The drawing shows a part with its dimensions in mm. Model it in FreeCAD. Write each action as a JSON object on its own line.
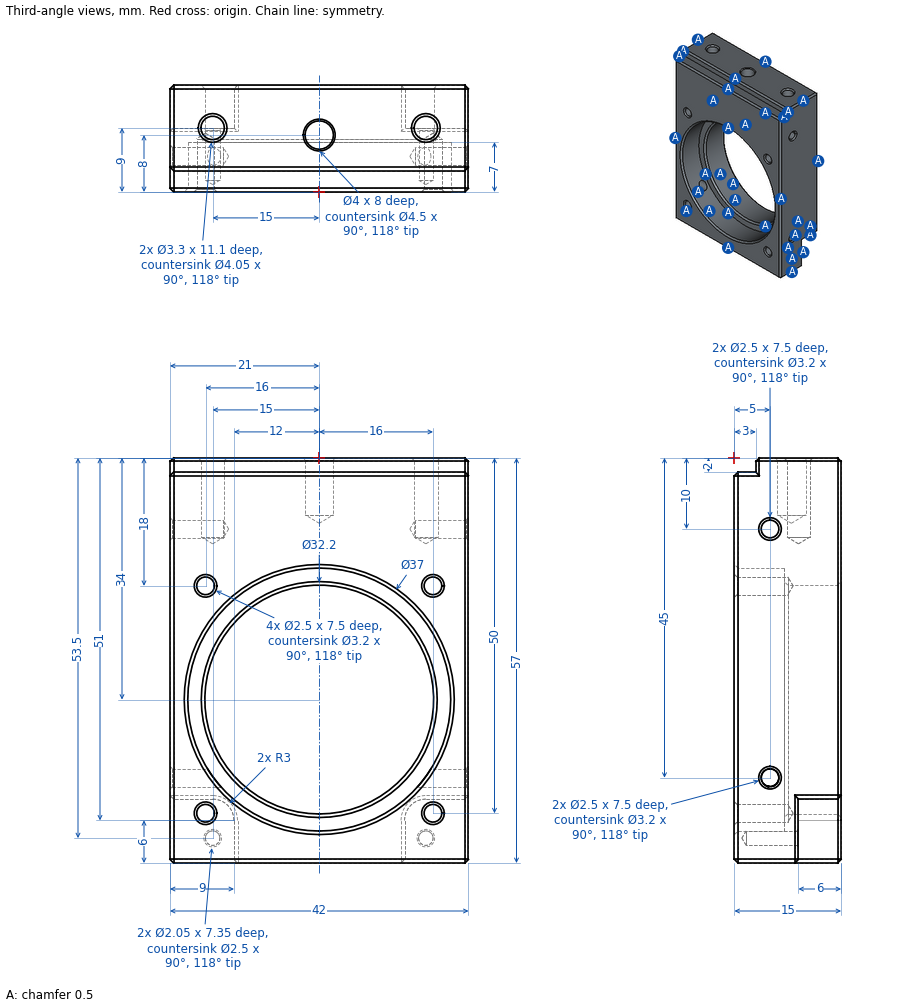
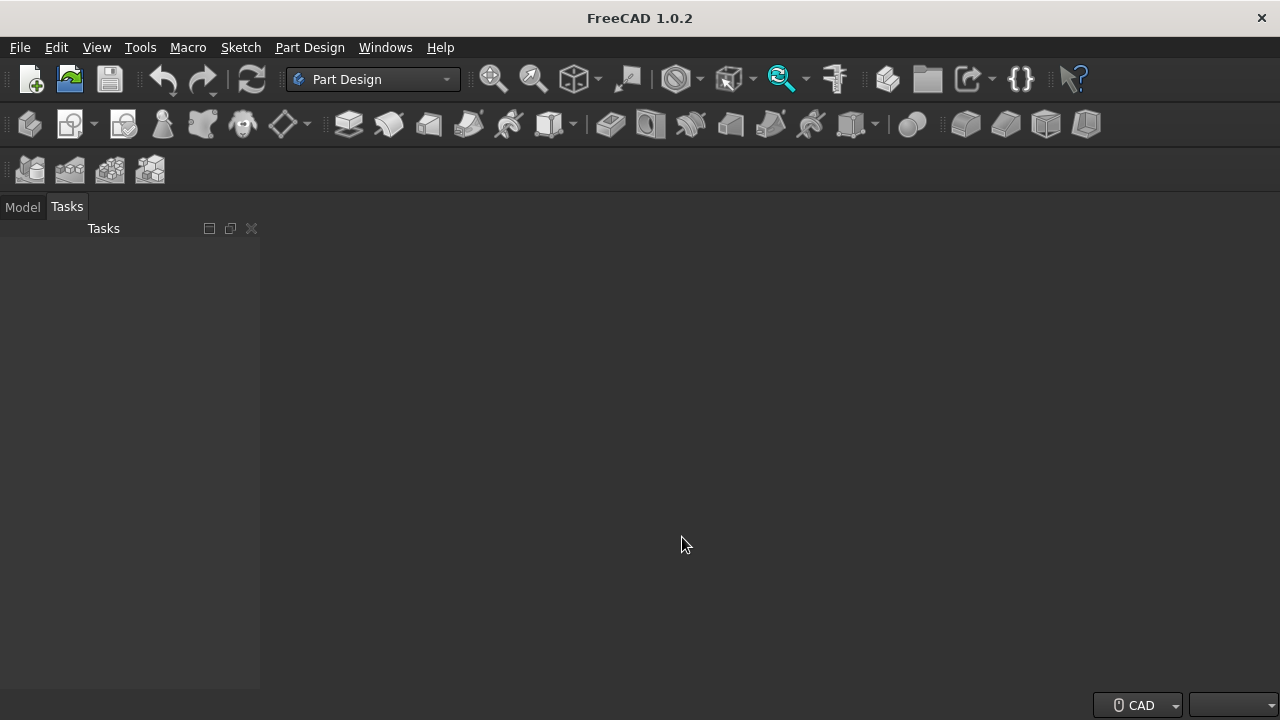
{"action": "key", "text": "ctrl+n"}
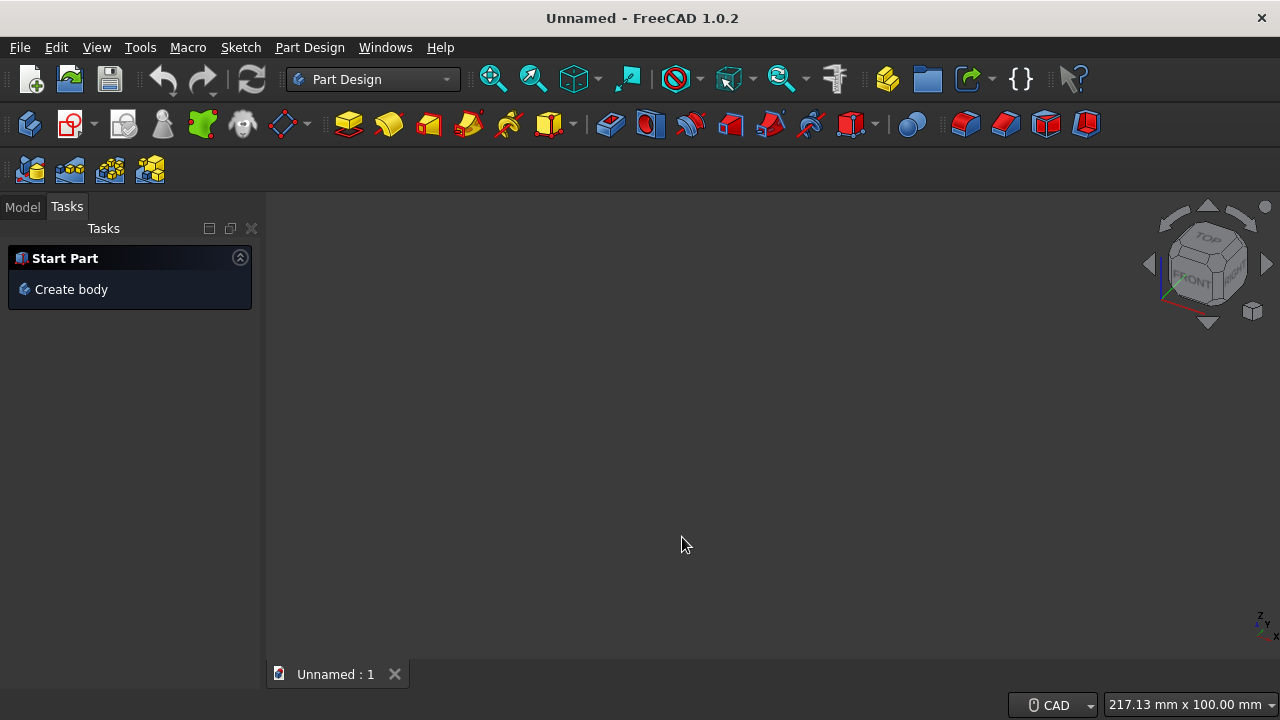
{"action": "left_click", "coordinate": [70, 124]}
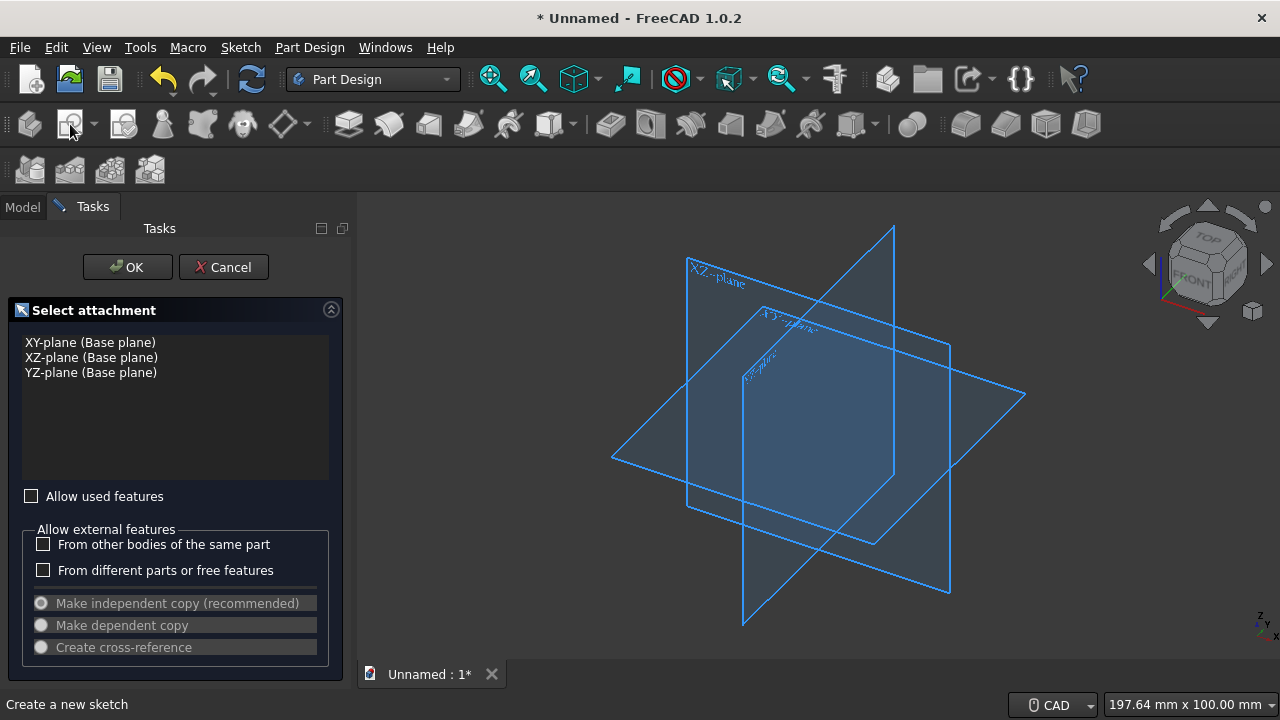
{"action": "left_click", "coordinate": [82, 358]}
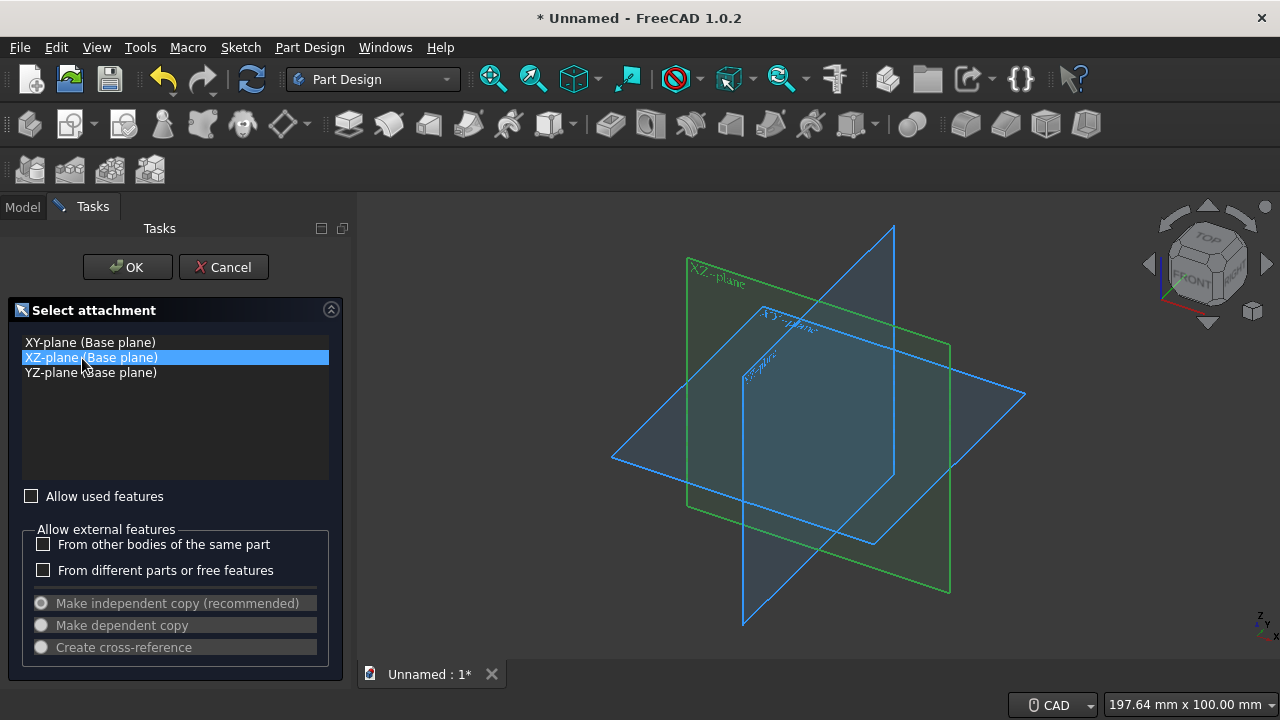
{"action": "left_click", "coordinate": [128, 267]}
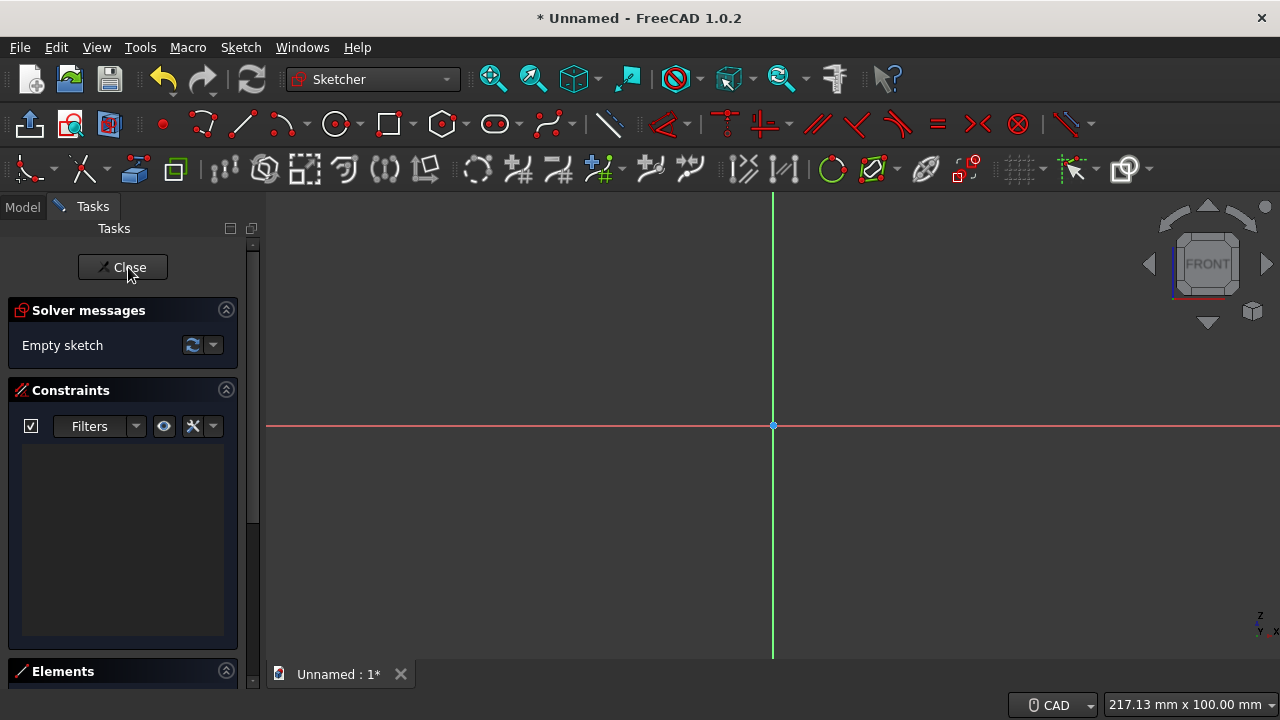
{"action": "scroll", "coordinate": [565, 220], "scroll_direction": "down", "scroll_amount": 2}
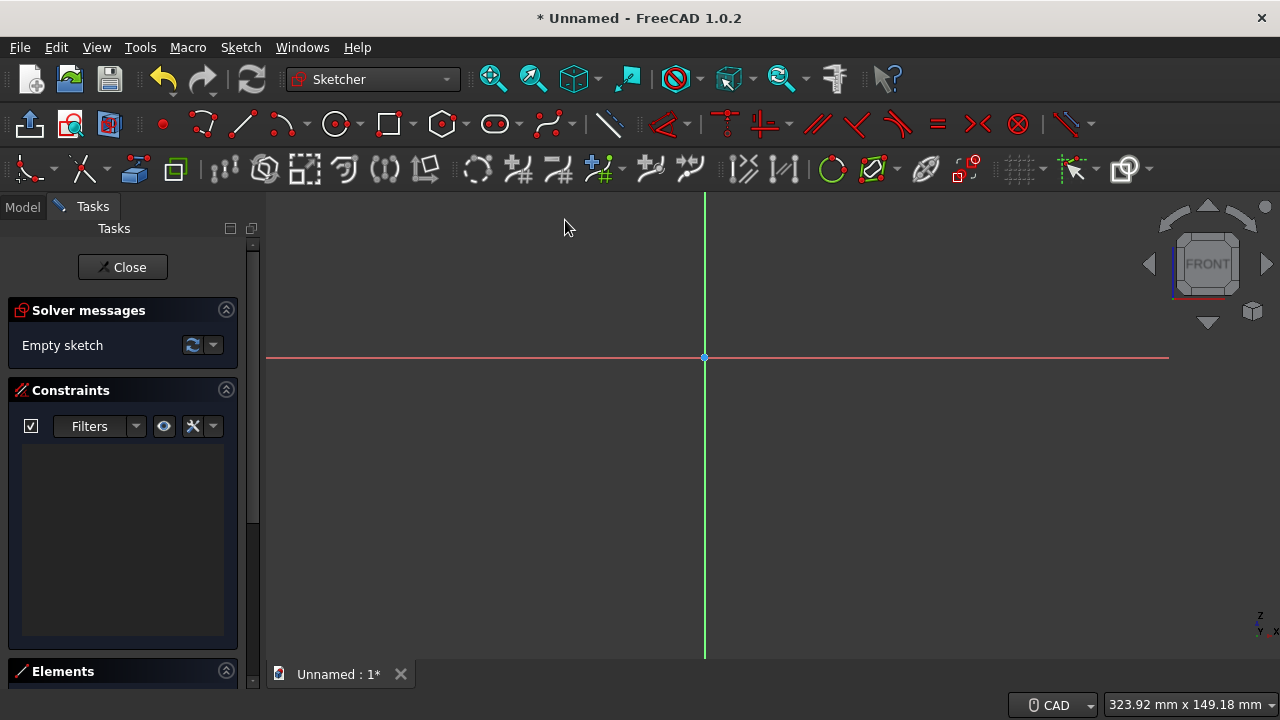
{"action": "scroll", "coordinate": [705, 491], "scroll_direction": "up", "scroll_amount": 2}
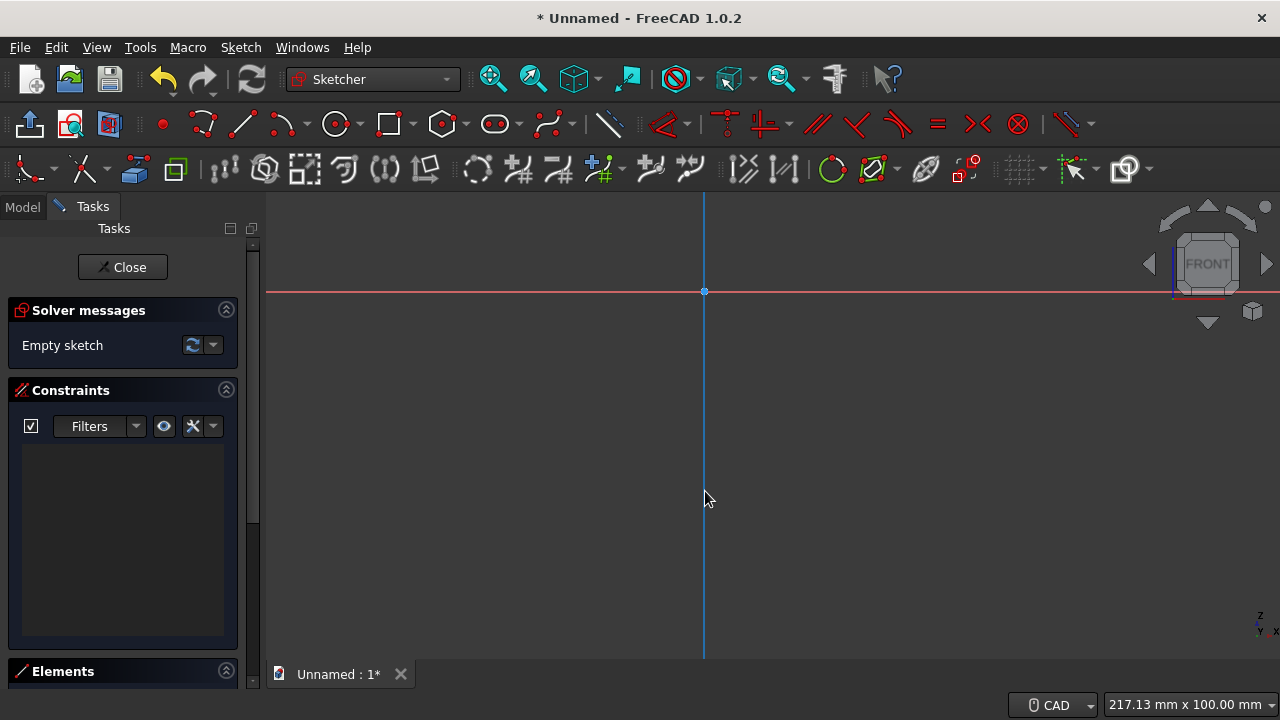
{"action": "left_click", "coordinate": [390, 124]}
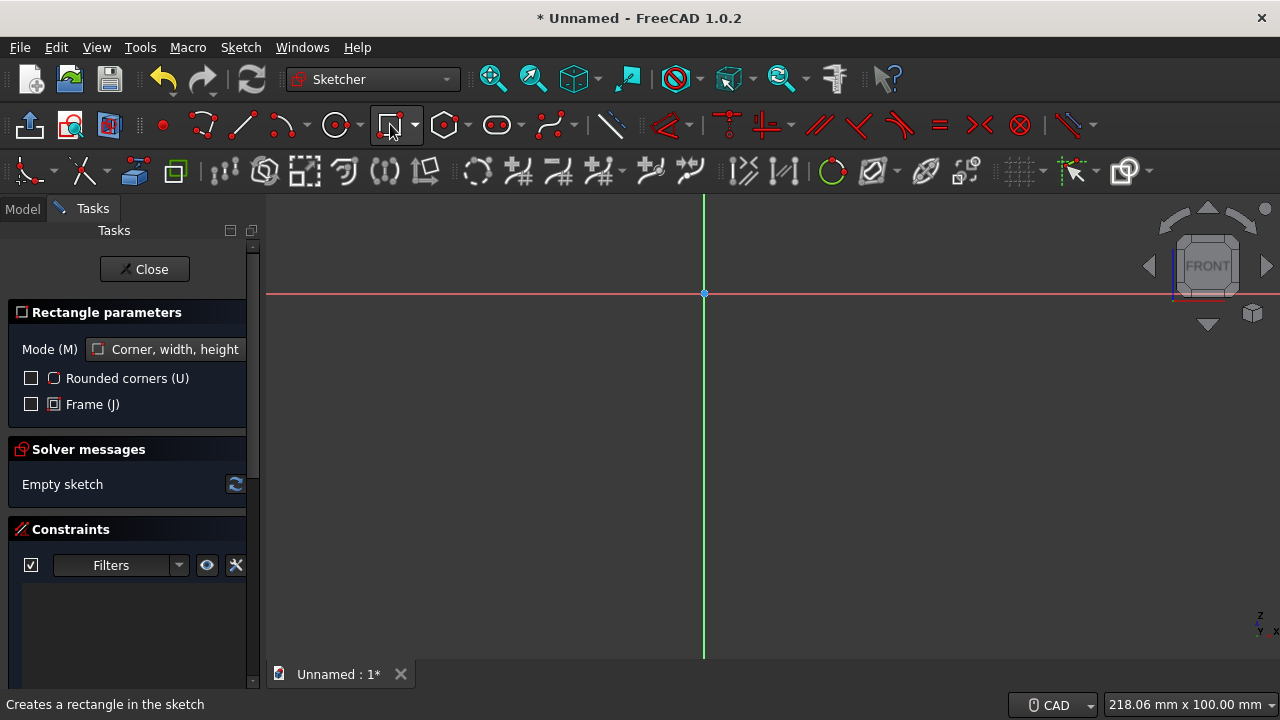
{"action": "left_click", "coordinate": [607, 294]}
{"action": "mouse_move", "coordinate": [802, 559]}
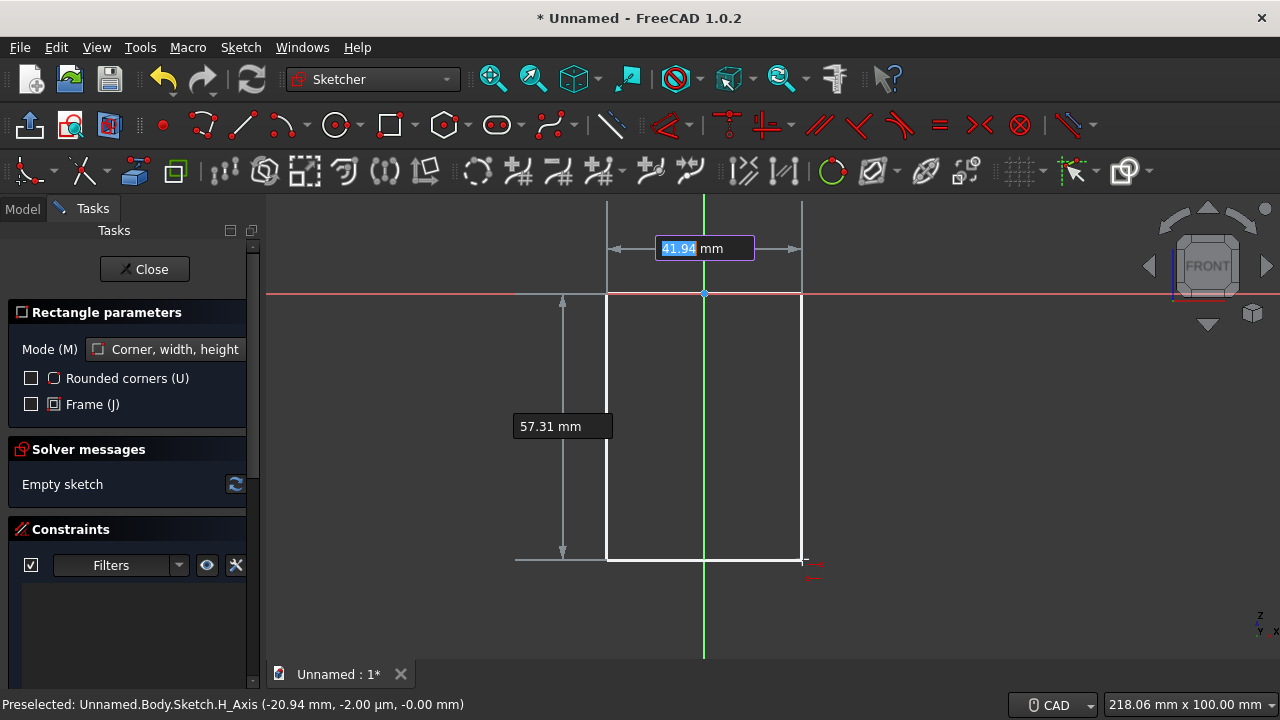
{"action": "type", "text": "42"}
{"action": "key", "text": "Tab"}
{"action": "type", "text": "57"}
{"action": "key", "text": "Return"}
{"action": "key", "text": "Escape"}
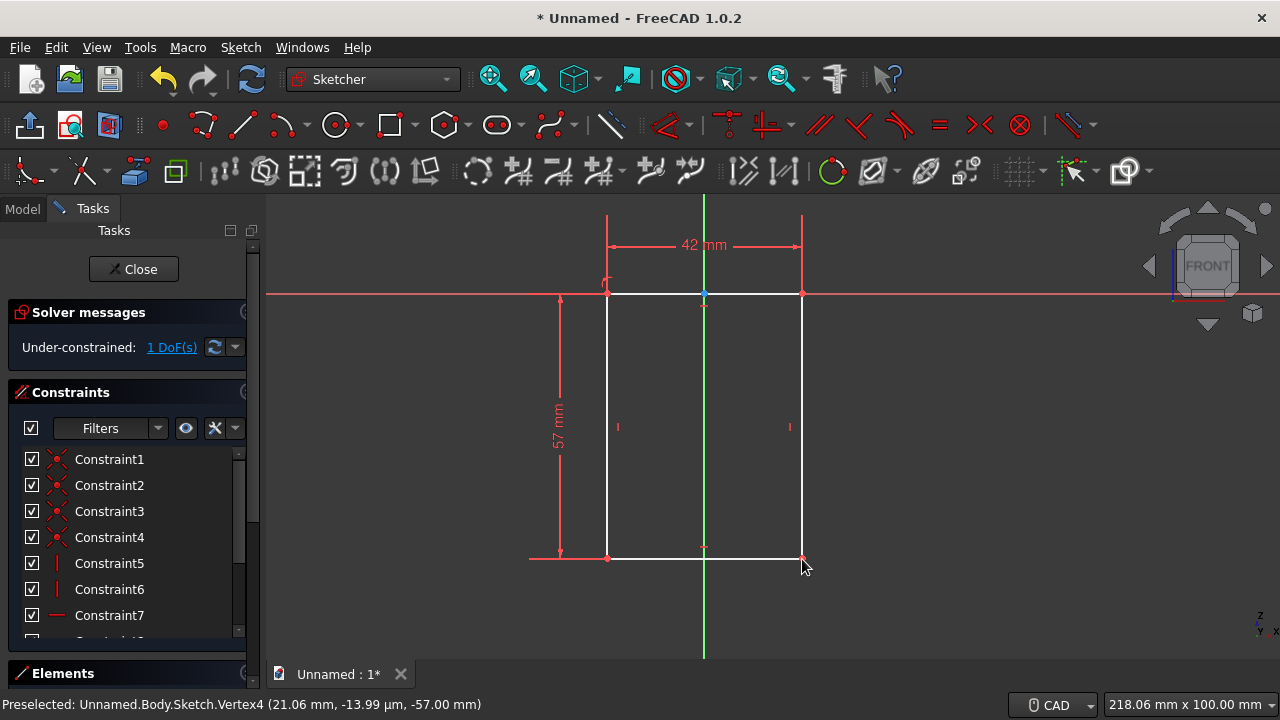
{"action": "key", "text": "d"}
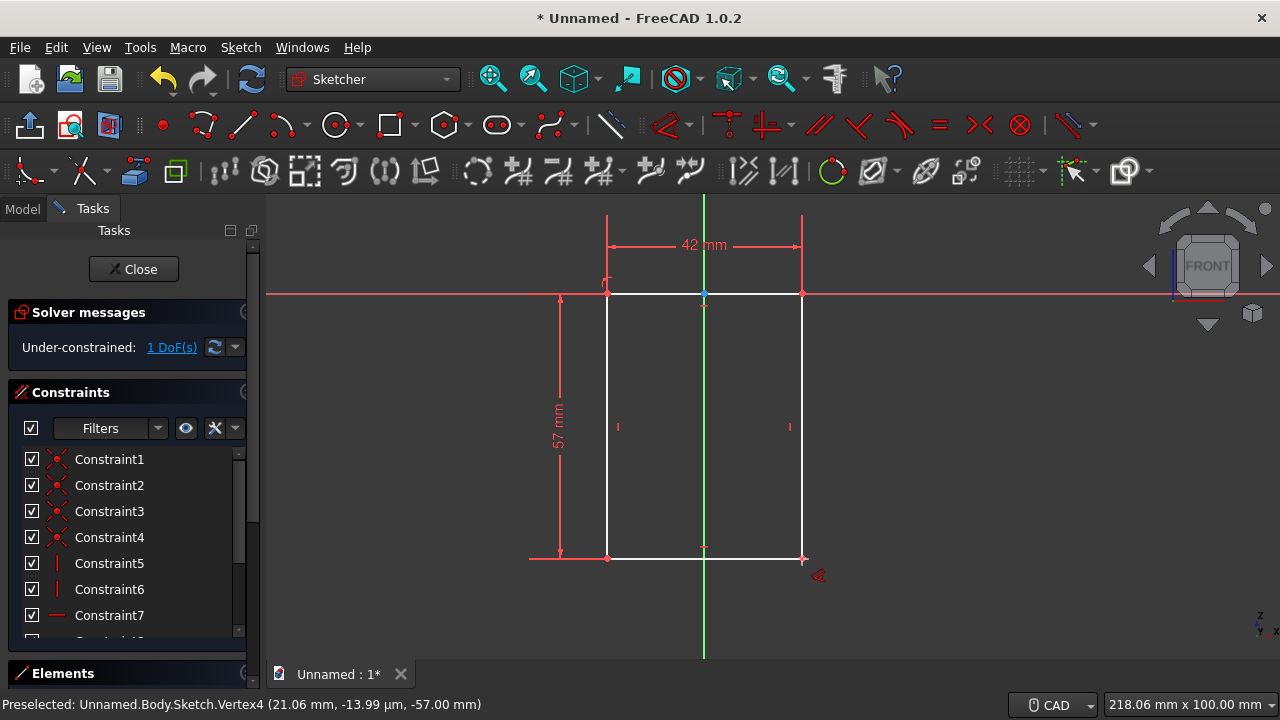
{"action": "left_click", "coordinate": [607, 294]}
{"action": "left_click", "coordinate": [656, 260]}